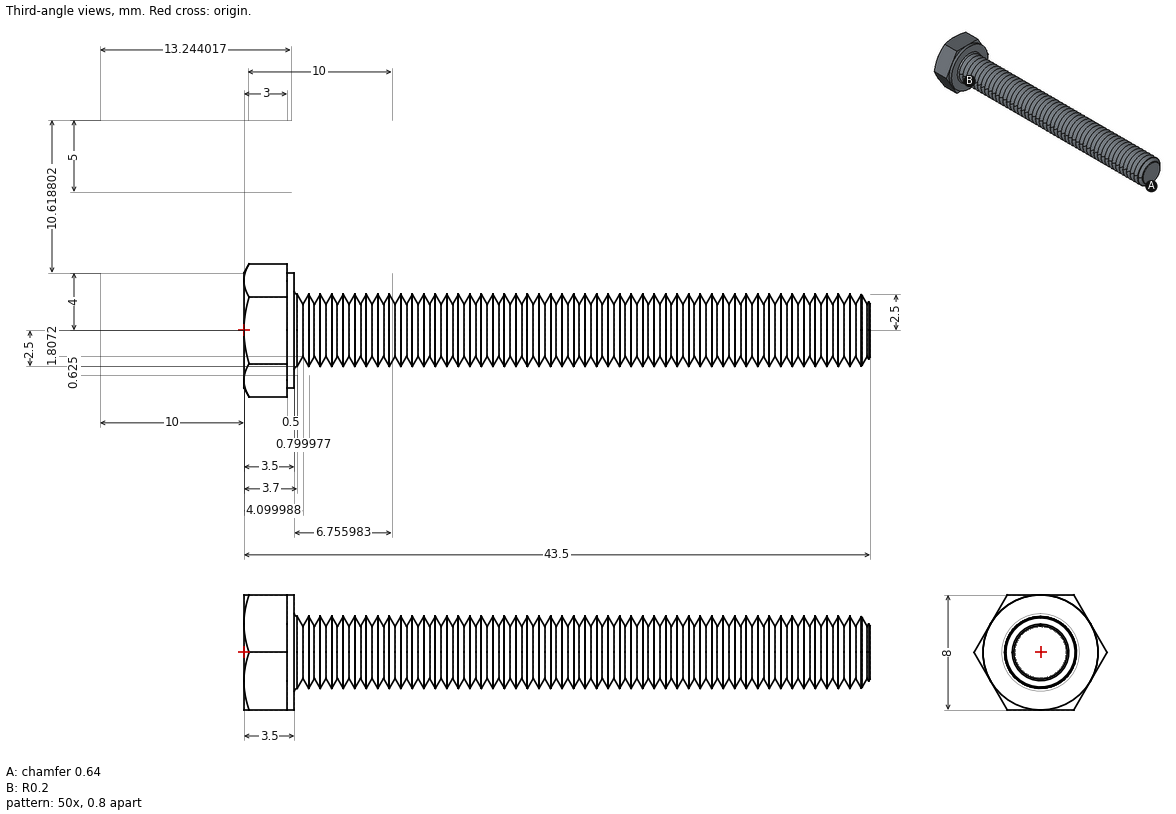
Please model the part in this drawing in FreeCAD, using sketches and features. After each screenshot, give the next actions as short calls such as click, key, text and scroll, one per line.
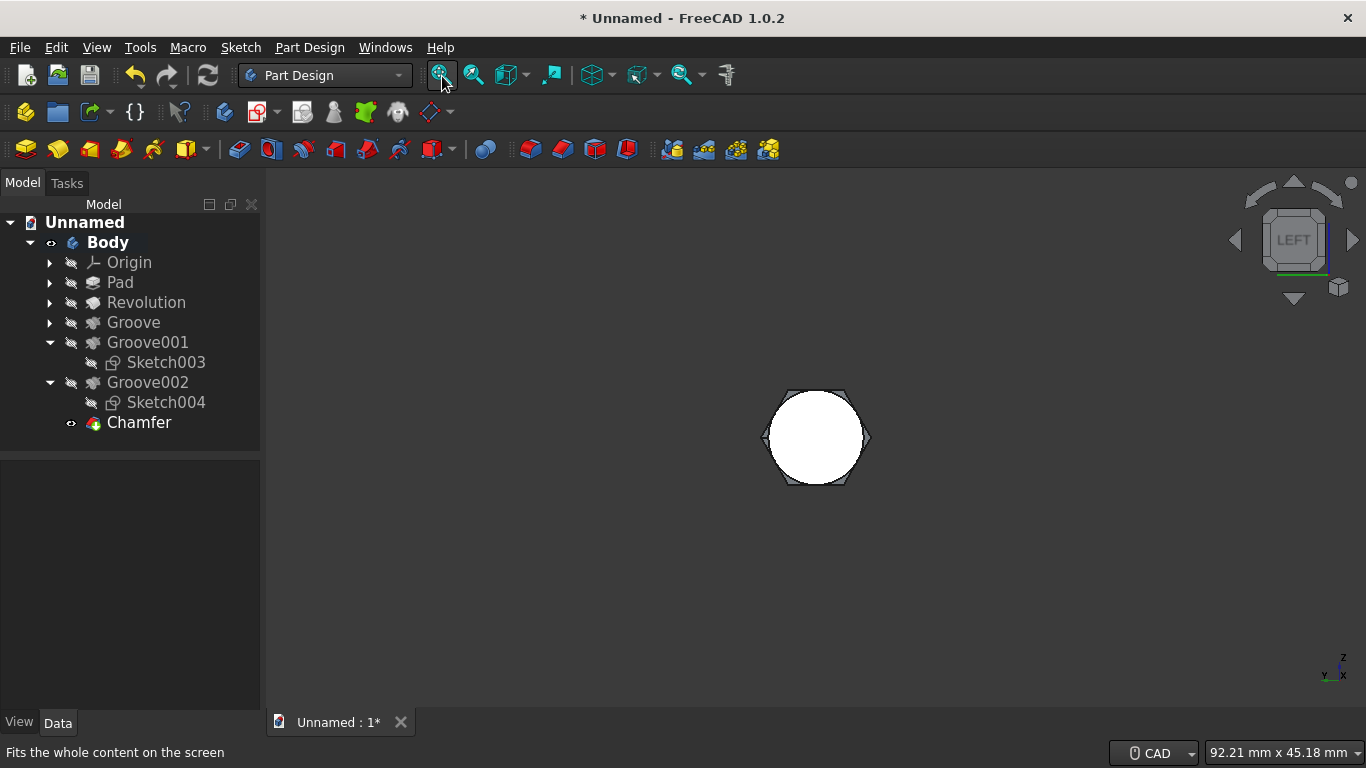
key(0)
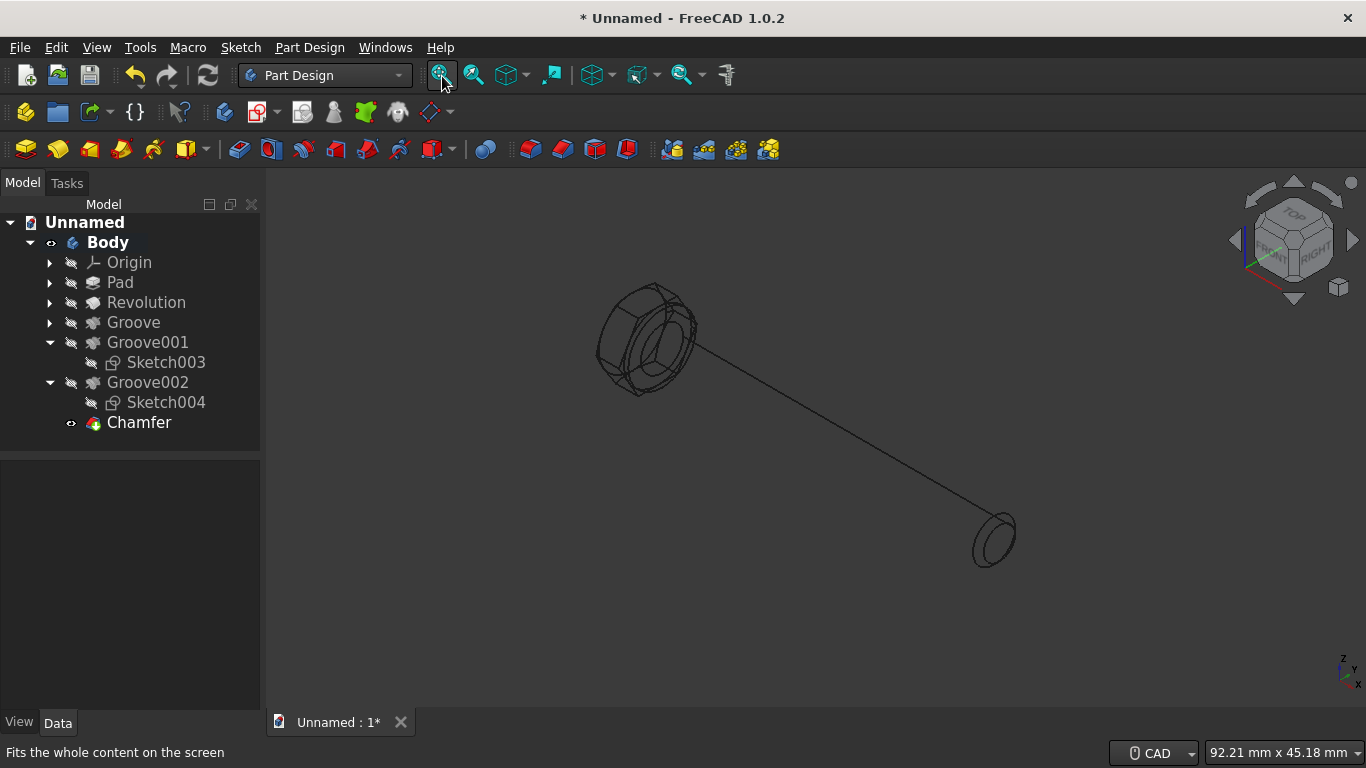
click(641, 360)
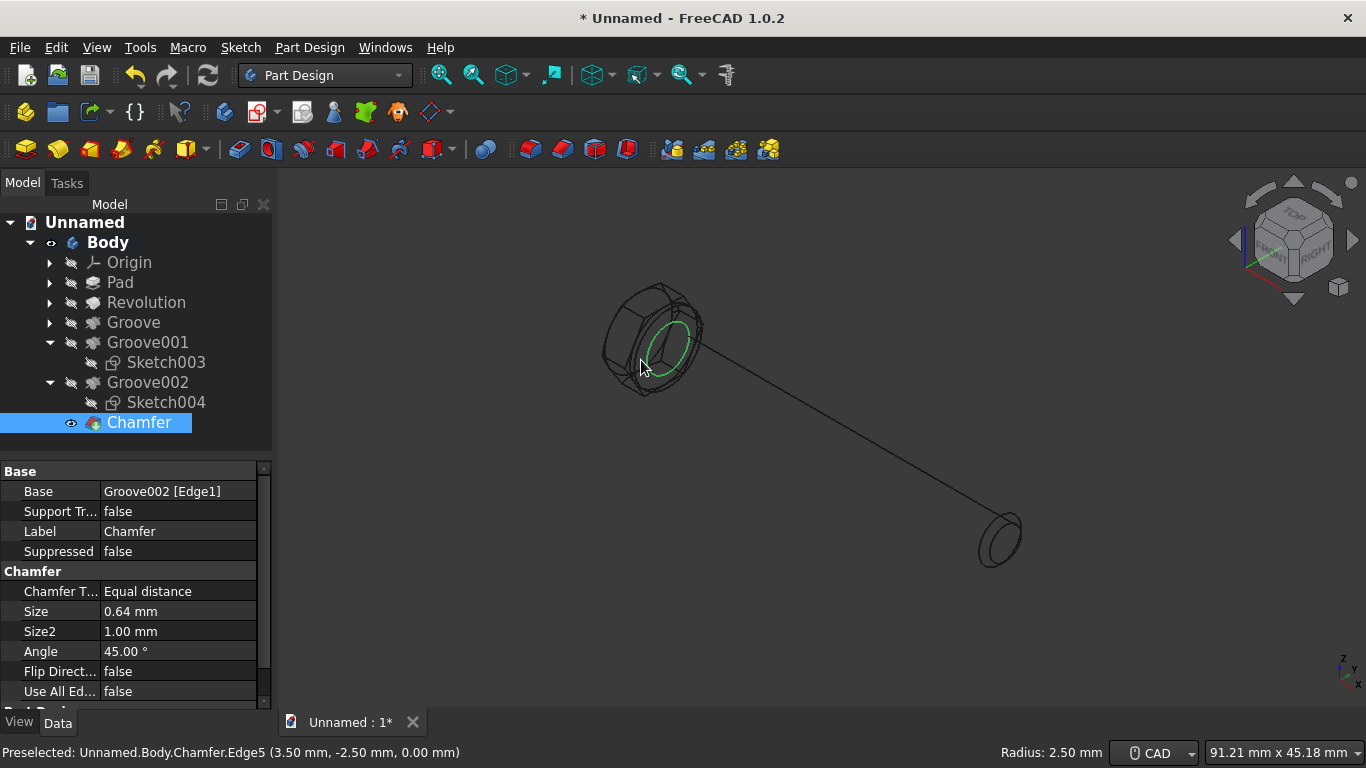
key(v)
key(1)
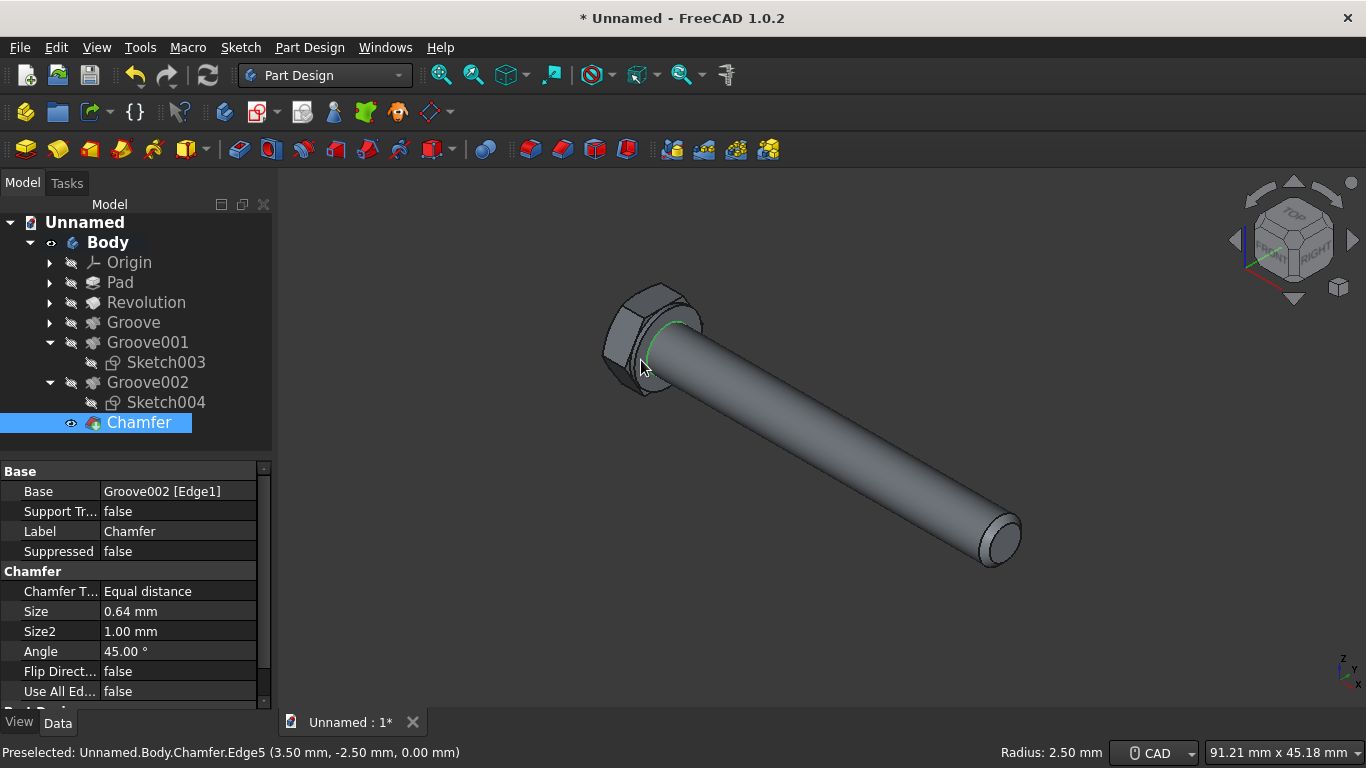
click(532, 150)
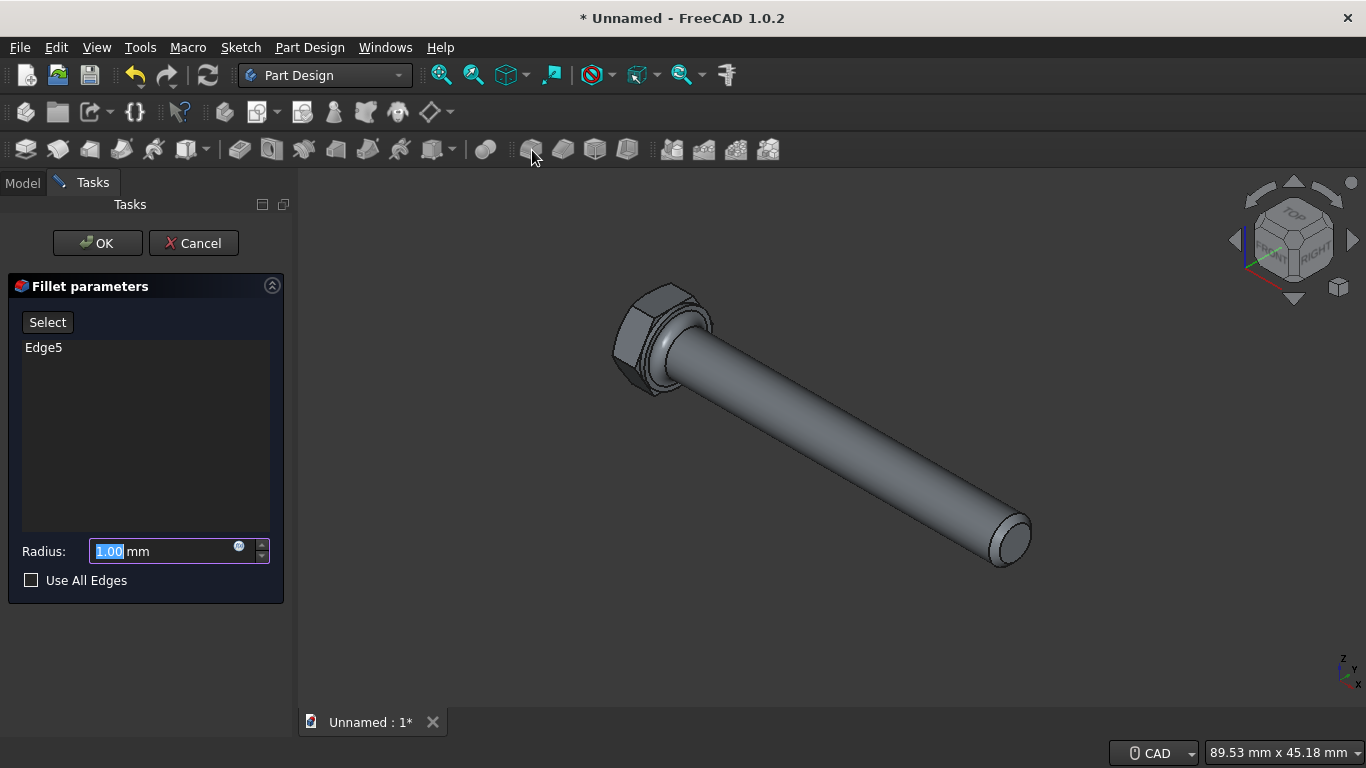
text(0.2)
key(Tab)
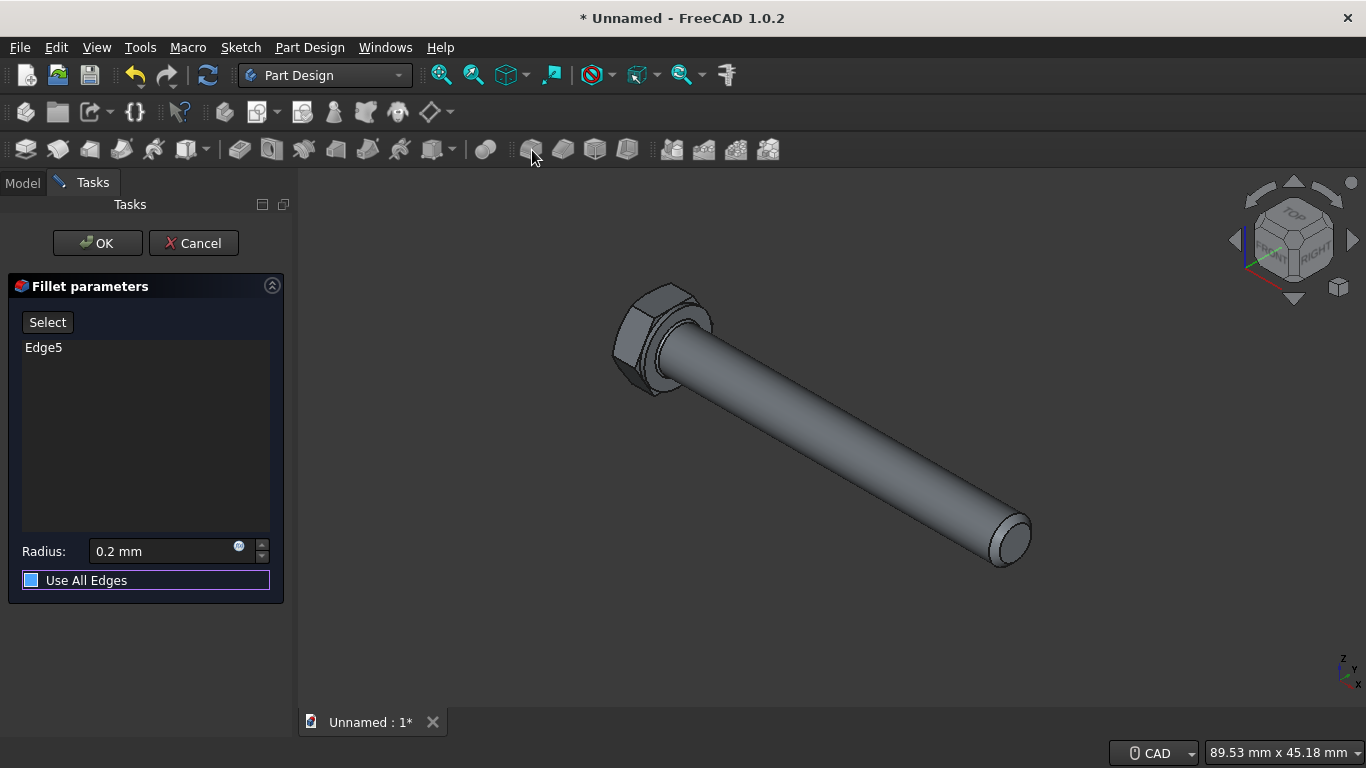
click(98, 243)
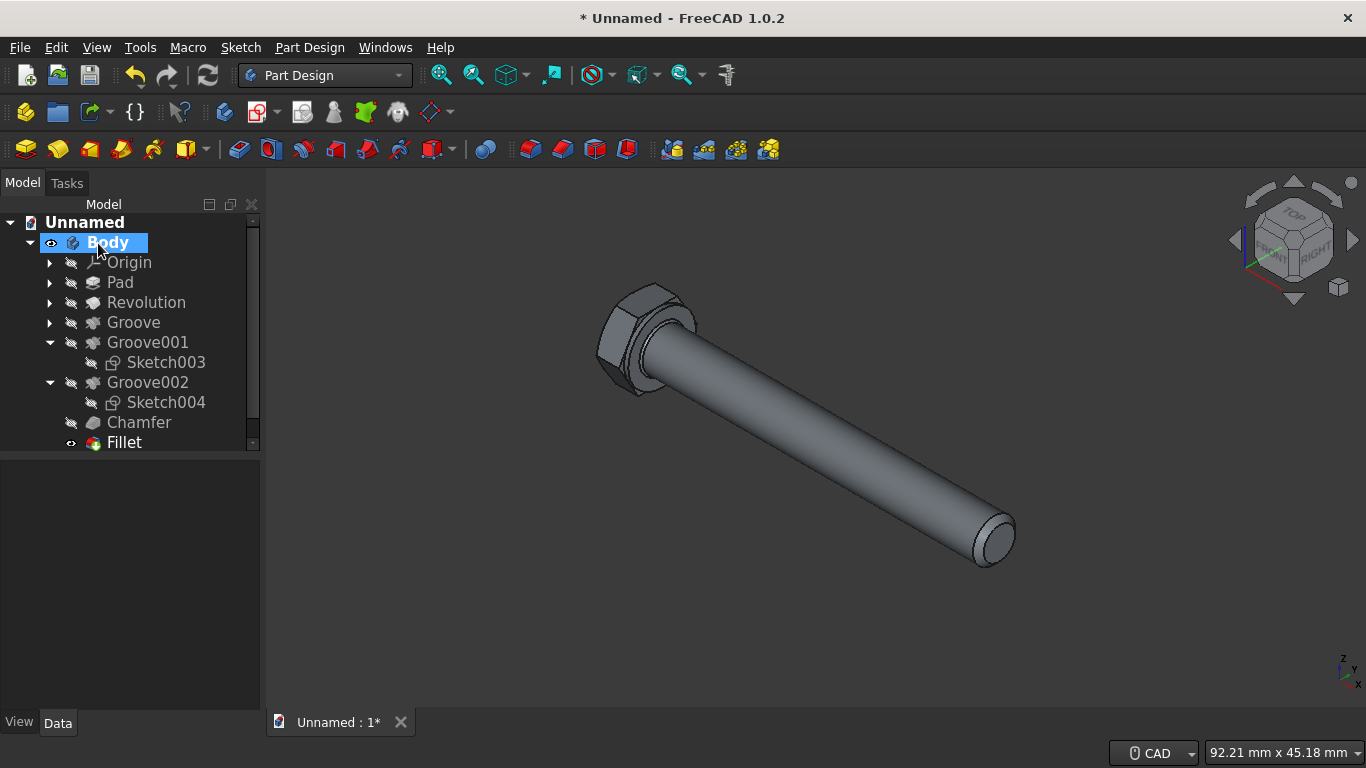
click(258, 112)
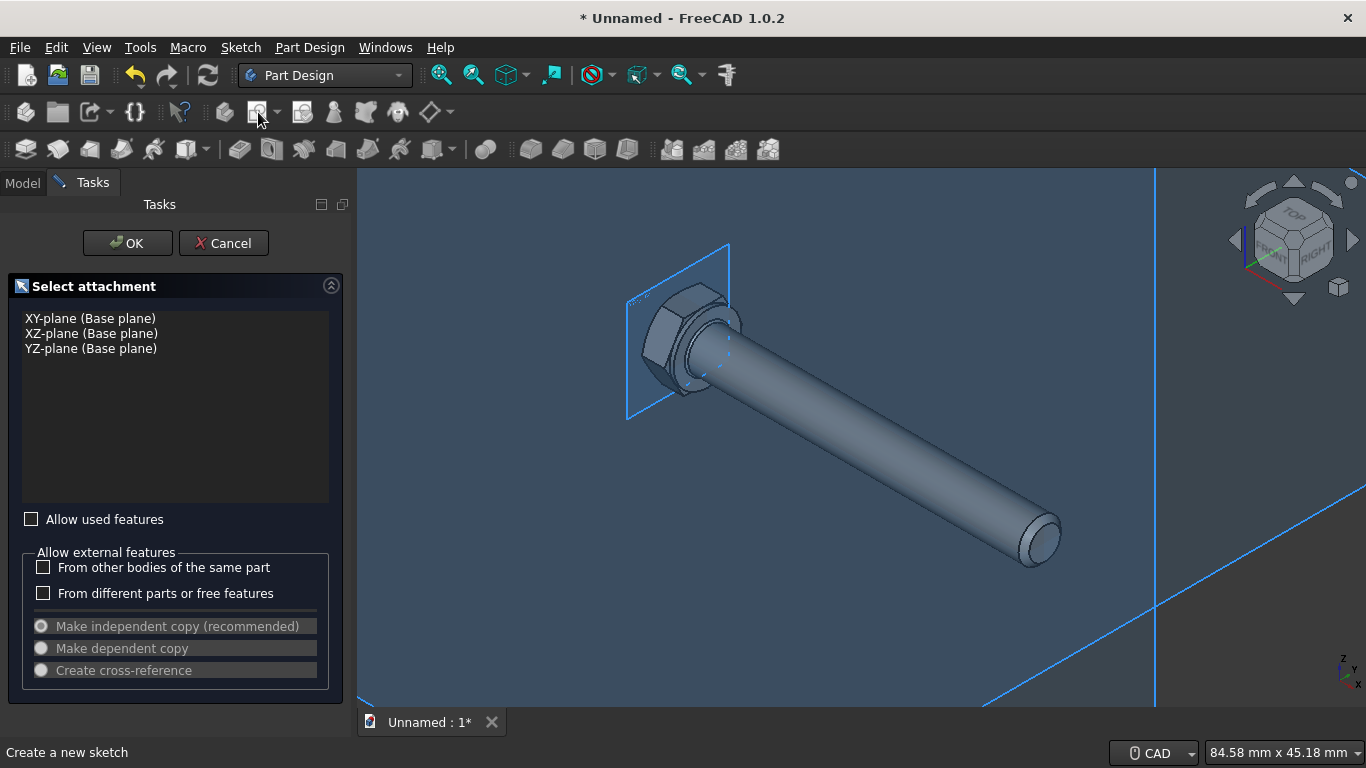
click(82, 318)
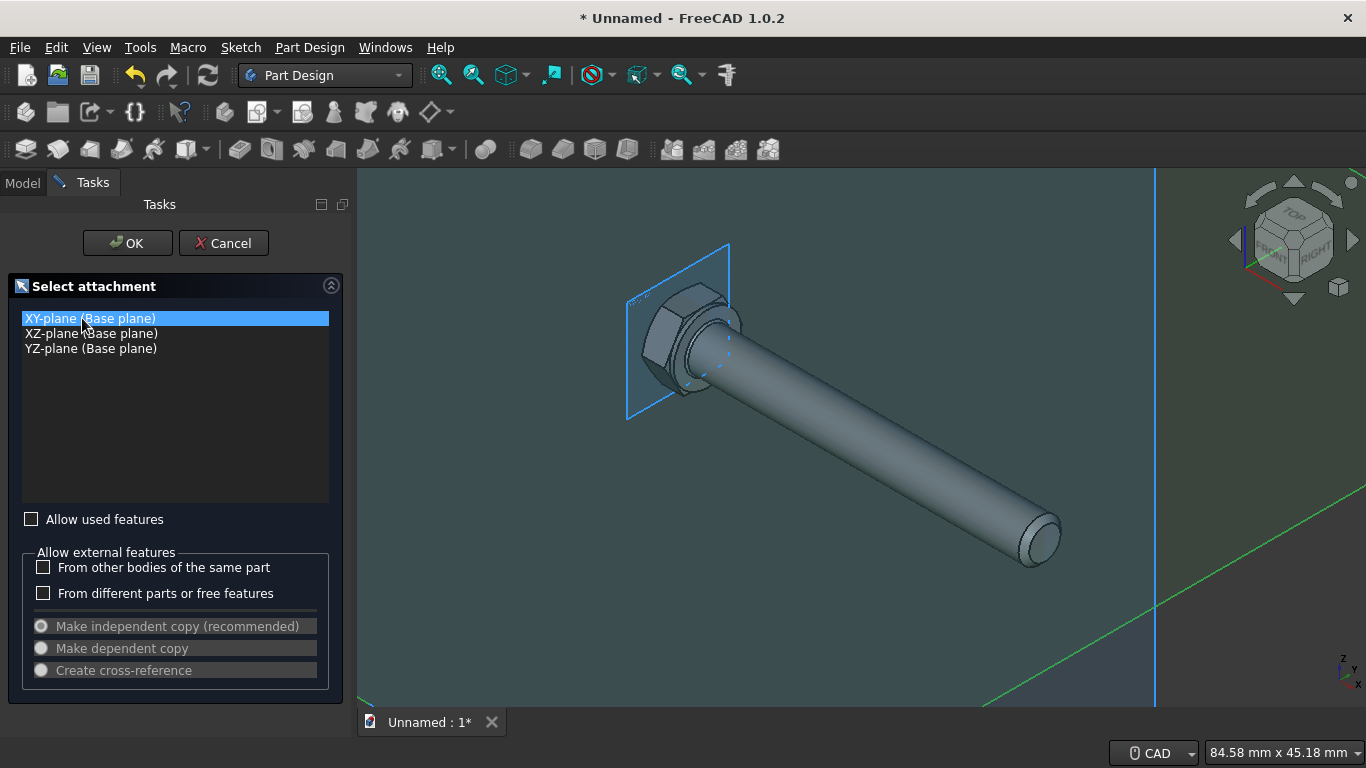
click(128, 243)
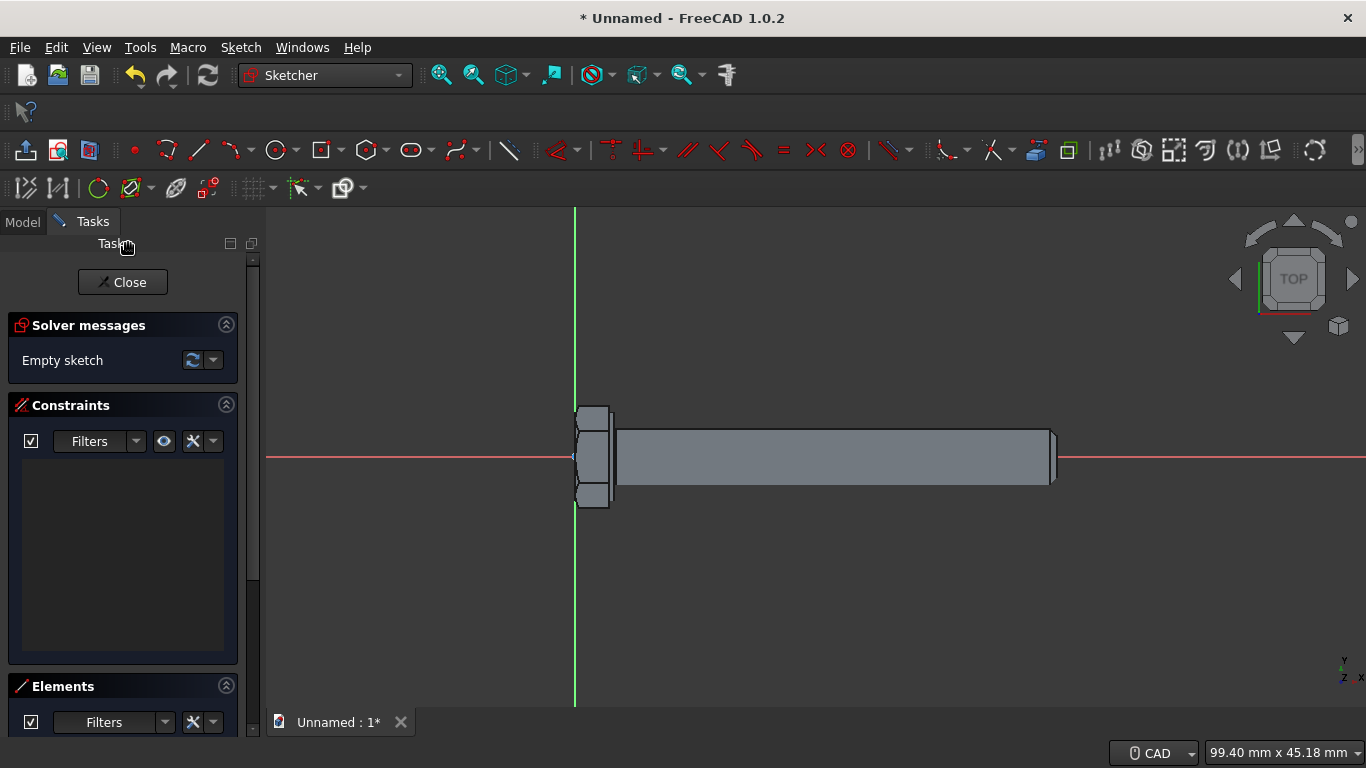
click(90, 150)